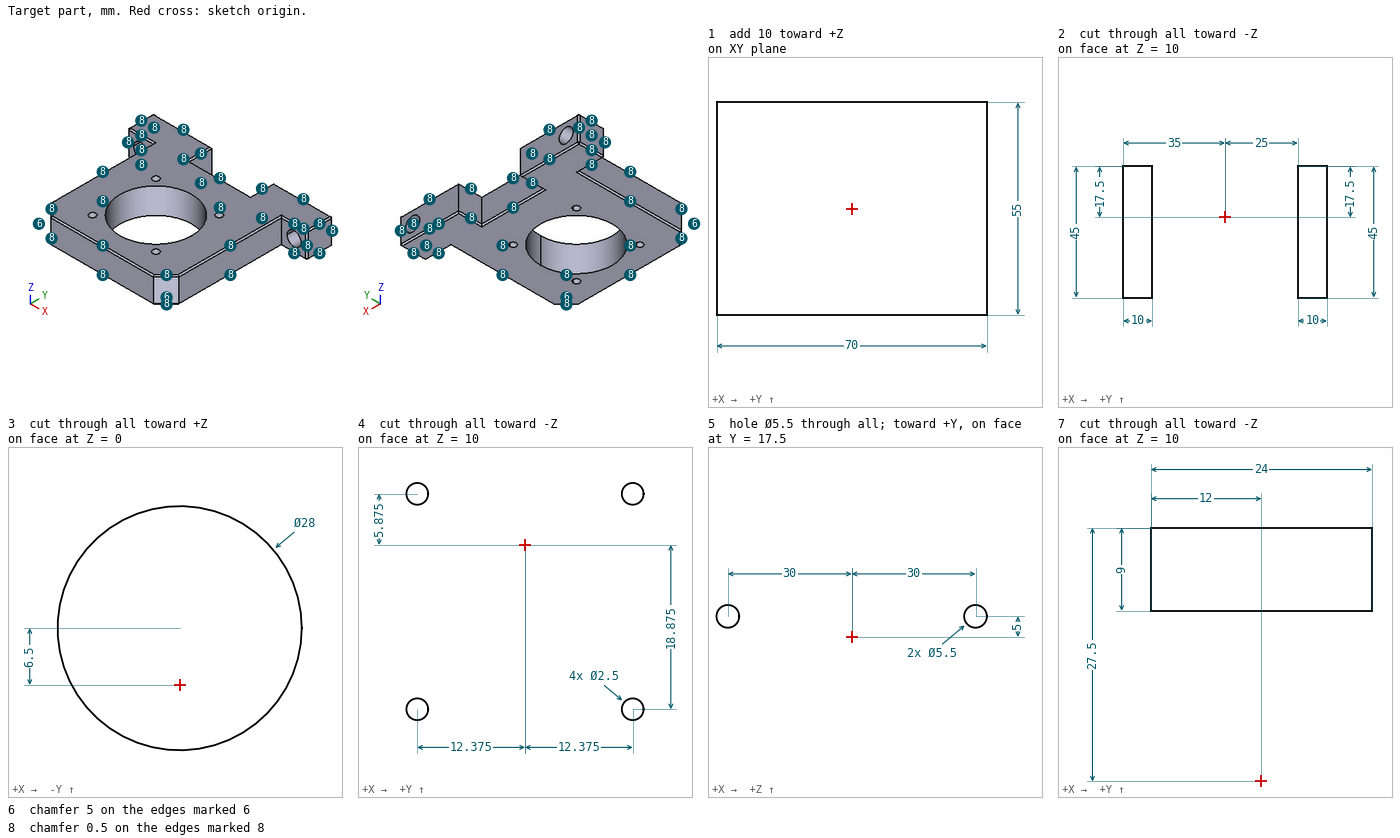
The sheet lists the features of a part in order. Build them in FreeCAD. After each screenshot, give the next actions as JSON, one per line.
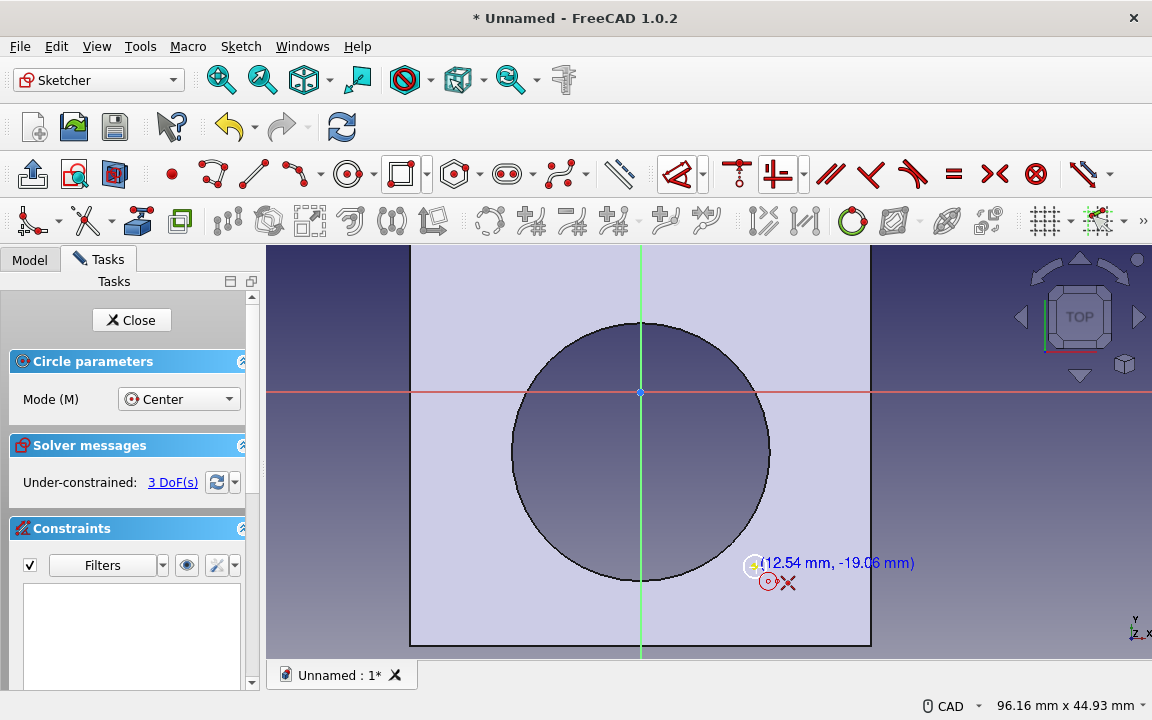
{"action": "scroll", "coordinate": [527, 566], "scroll_direction": "up", "scroll_amount": 4}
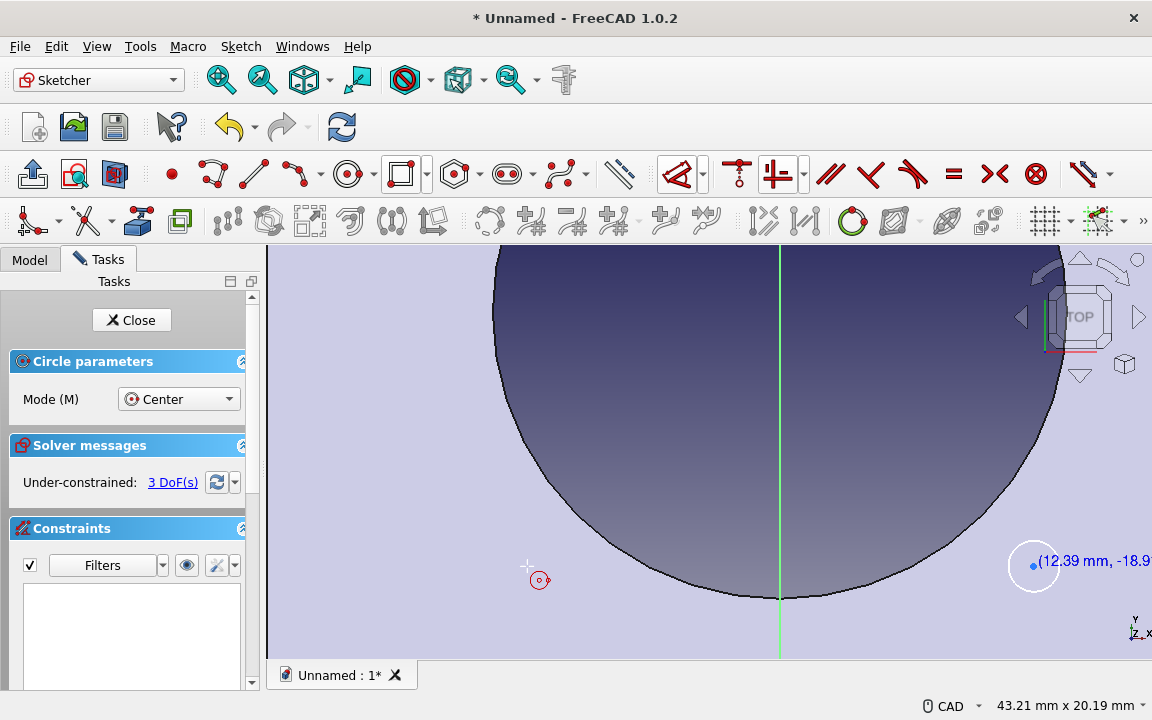
{"action": "left_click", "coordinate": [526, 565]}
{"action": "left_click", "coordinate": [544, 547]}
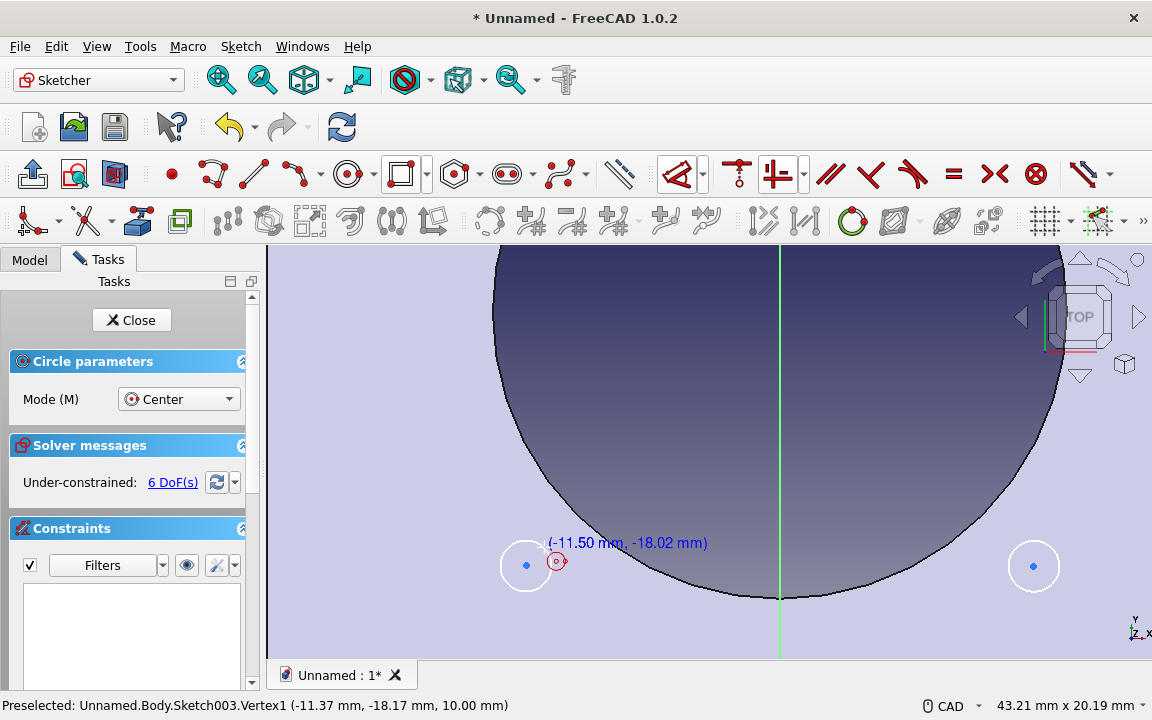
{"action": "scroll", "coordinate": [527, 566], "scroll_direction": "down", "scroll_amount": 4}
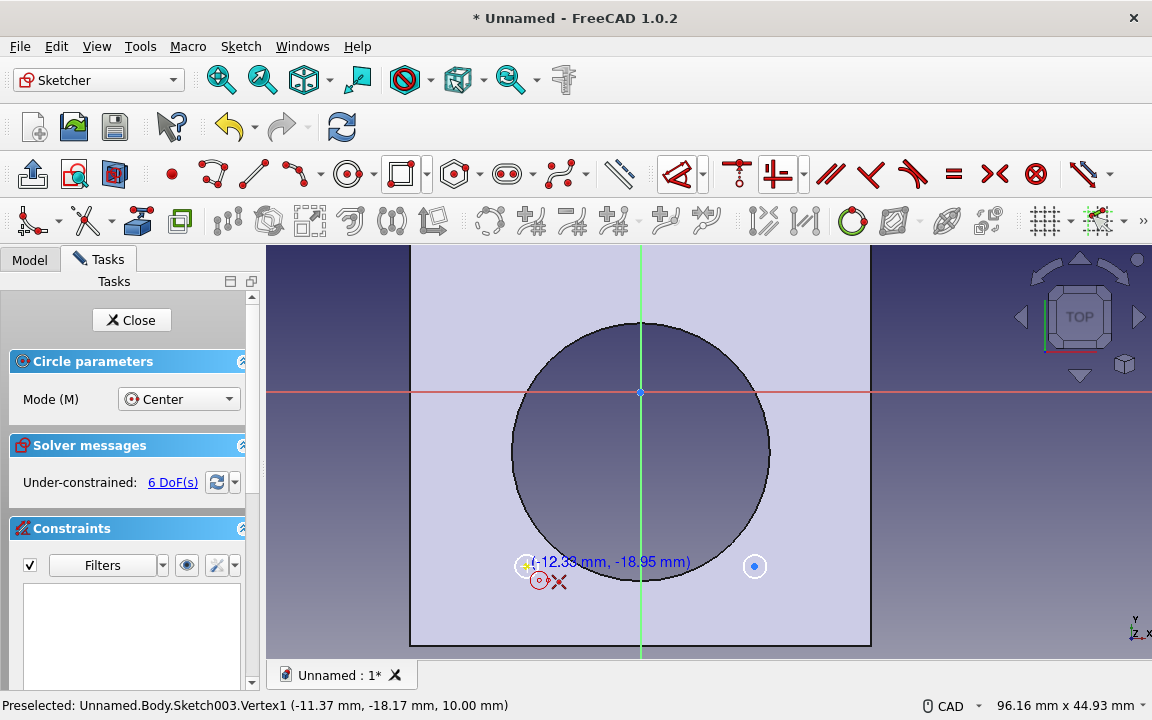
{"action": "scroll", "coordinate": [527, 338], "scroll_direction": "up", "scroll_amount": 4}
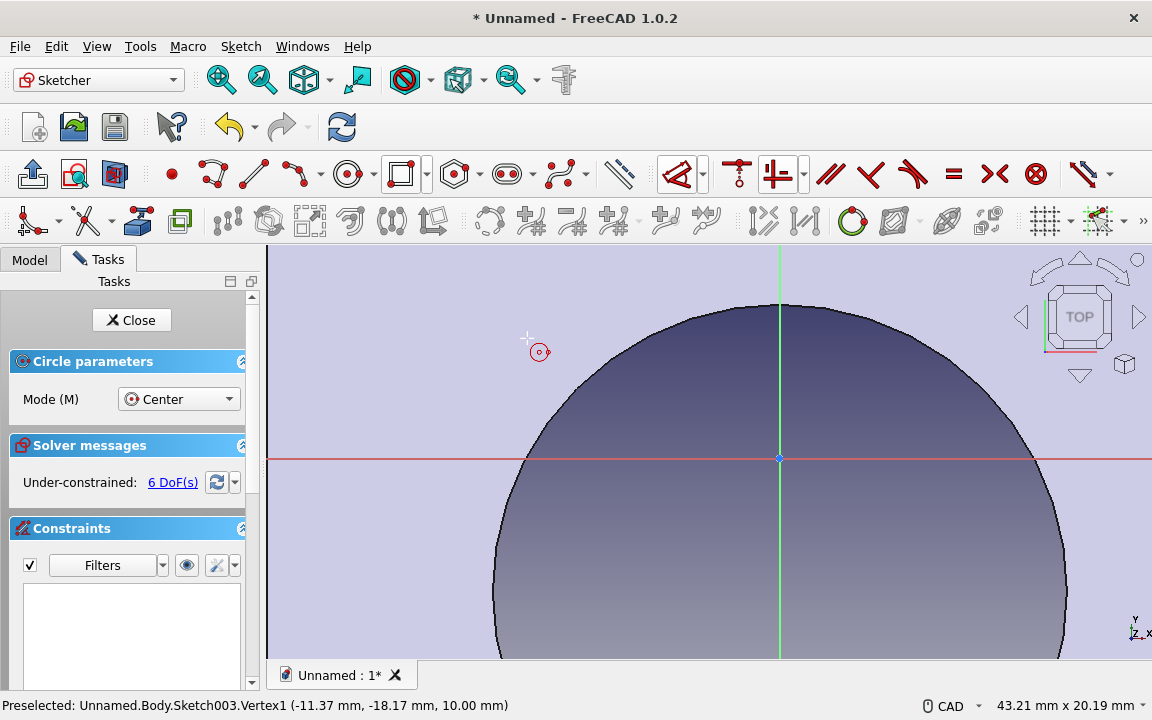
{"action": "left_click", "coordinate": [526, 338]}
{"action": "left_click", "coordinate": [544, 320]}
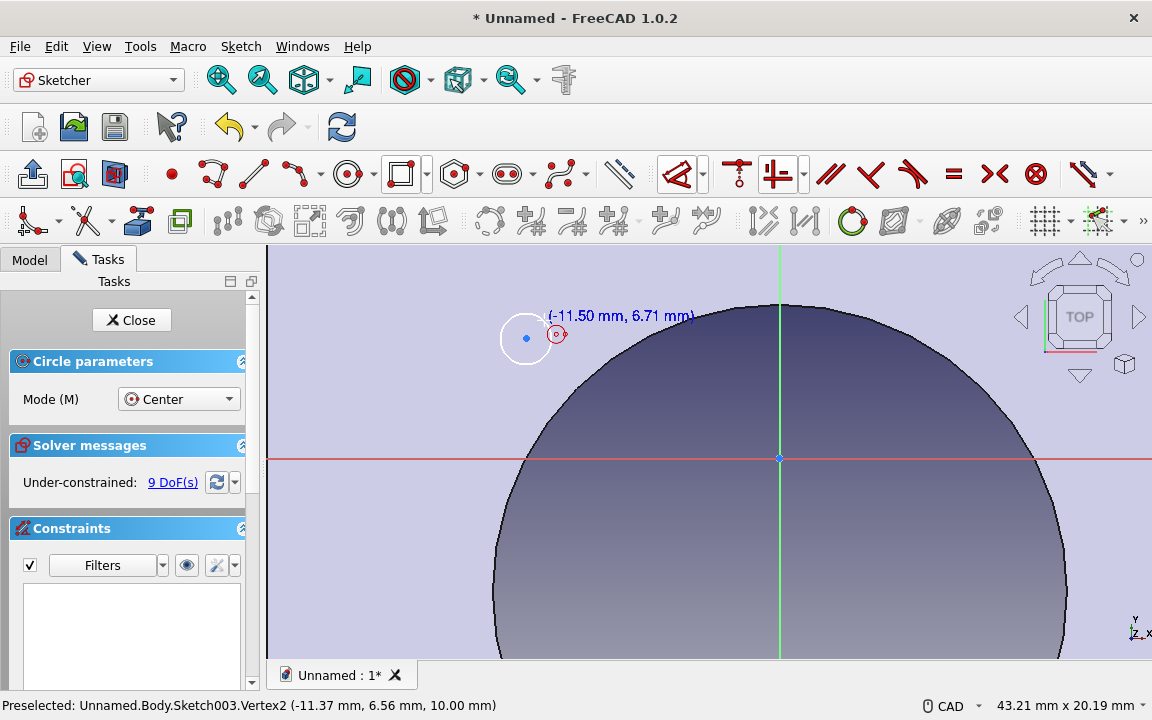
{"action": "scroll", "coordinate": [527, 338], "scroll_direction": "down", "scroll_amount": 4}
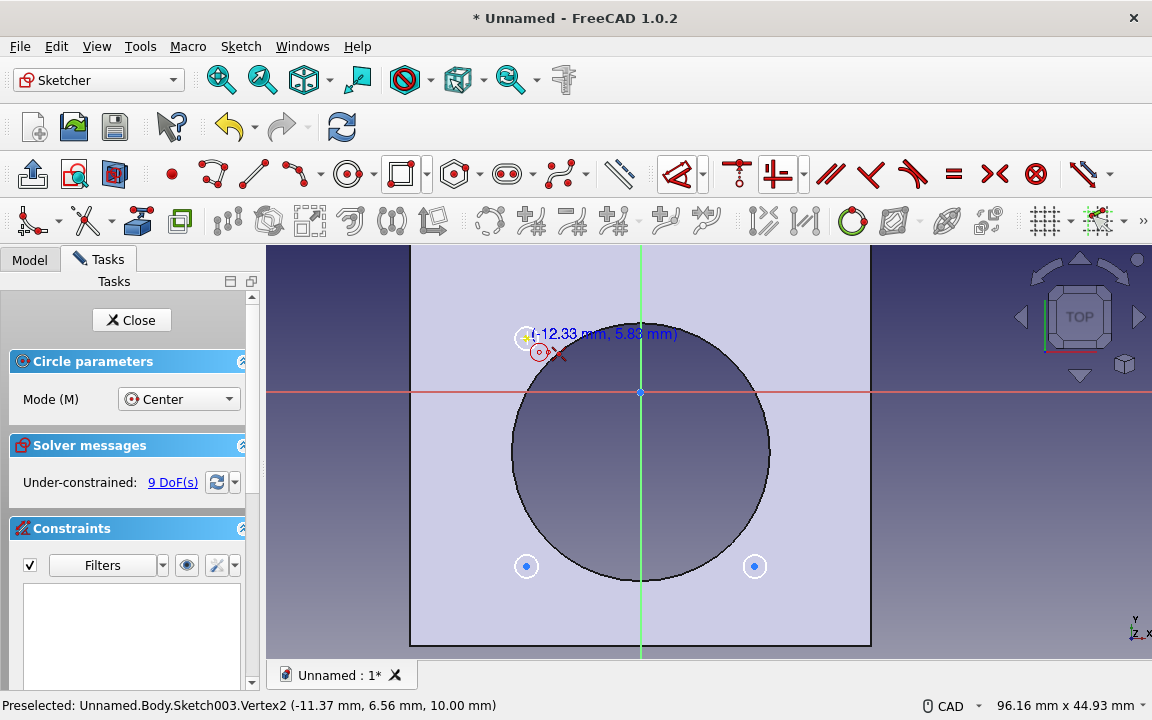
{"action": "scroll", "coordinate": [755, 338], "scroll_direction": "up", "scroll_amount": 4}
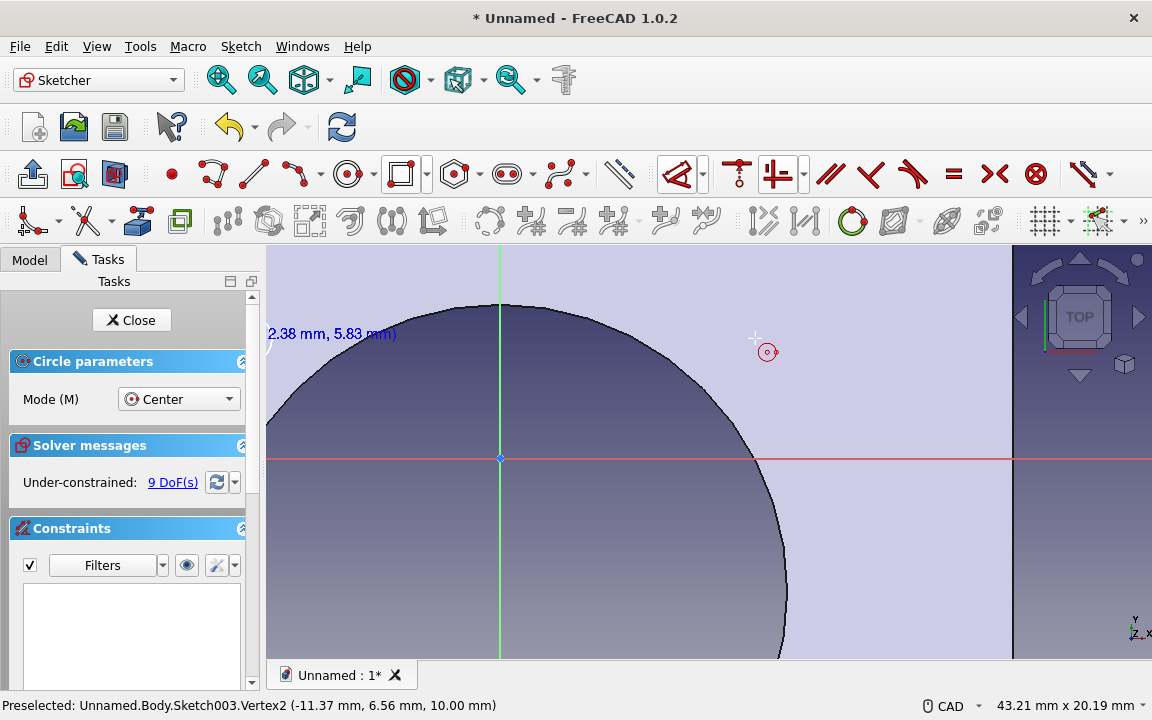
{"action": "left_click", "coordinate": [754, 338]}
{"action": "left_click", "coordinate": [772, 320]}
{"action": "key", "text": "Escape"}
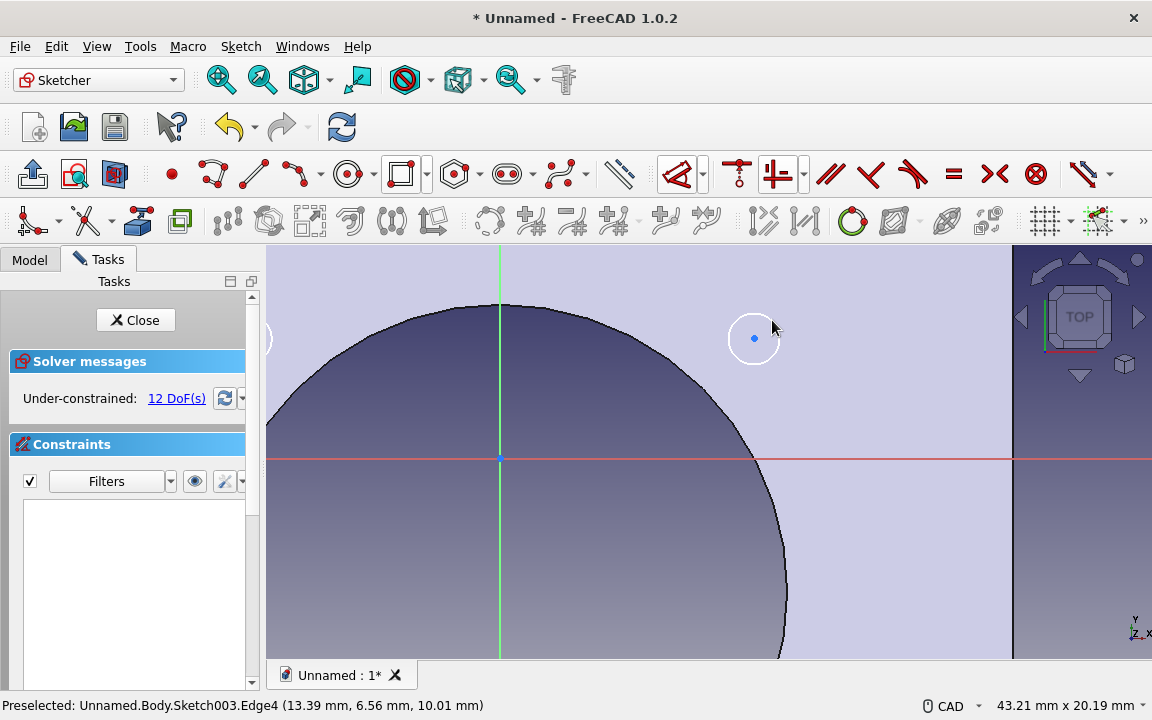
{"action": "scroll", "coordinate": [755, 338], "scroll_direction": "down", "scroll_amount": 4}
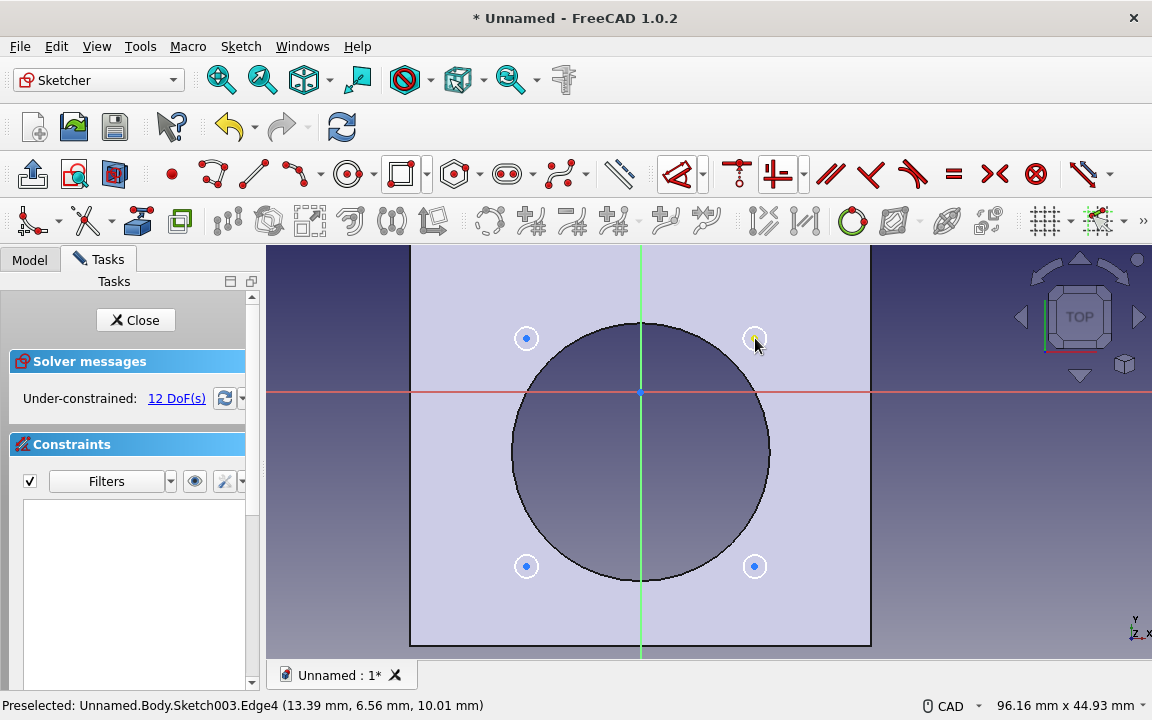
{"action": "left_click", "coordinate": [763, 558]}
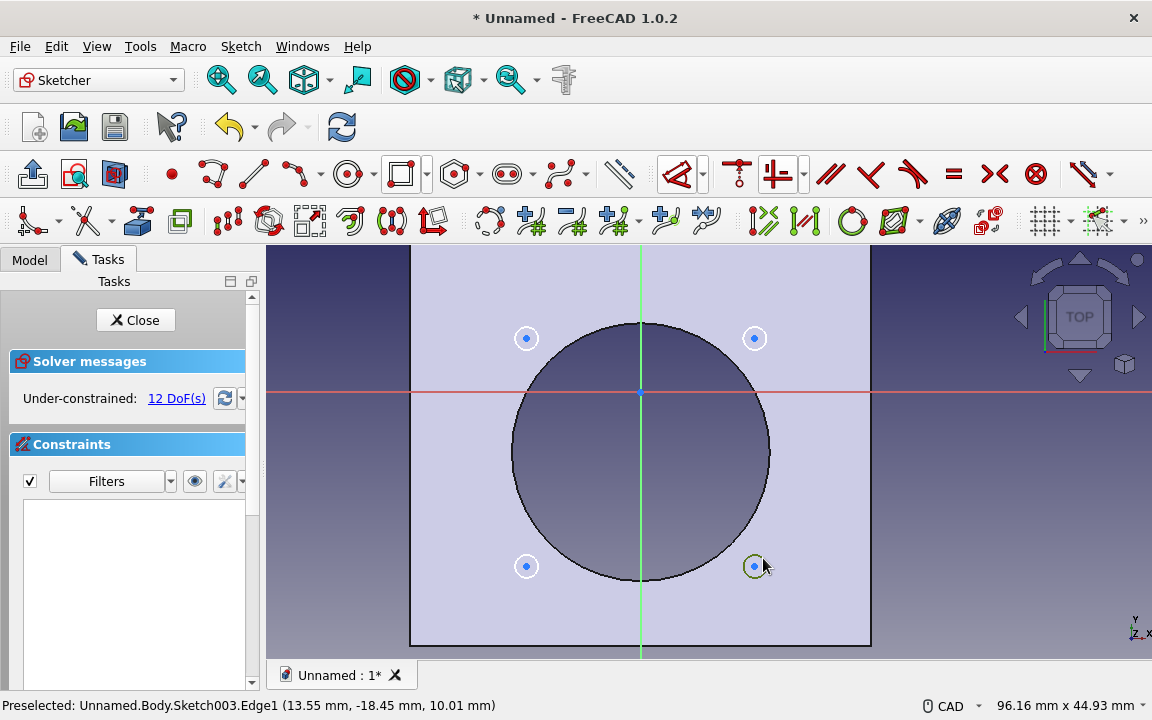
{"action": "left_click", "coordinate": [535, 558]}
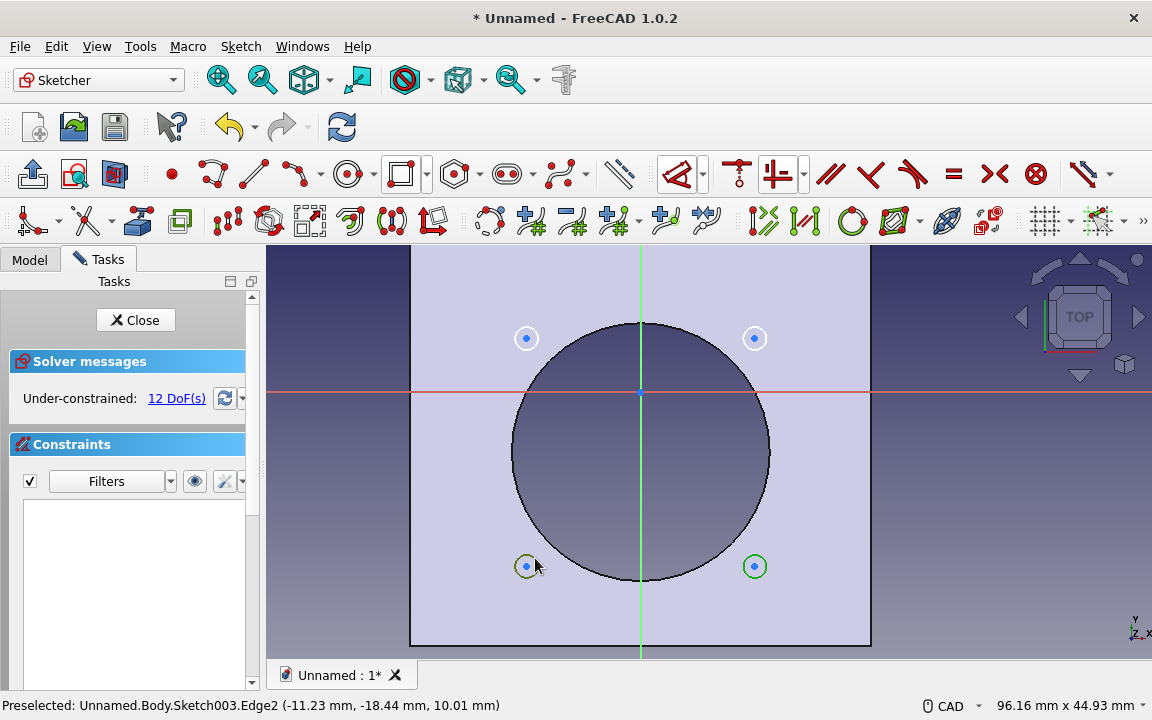
{"action": "left_click", "coordinate": [535, 330]}